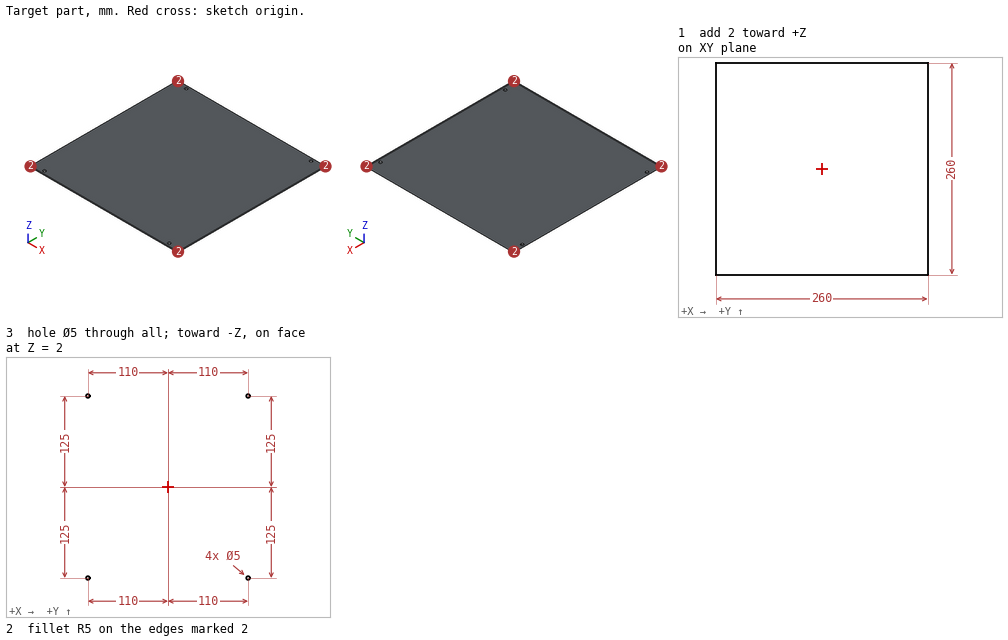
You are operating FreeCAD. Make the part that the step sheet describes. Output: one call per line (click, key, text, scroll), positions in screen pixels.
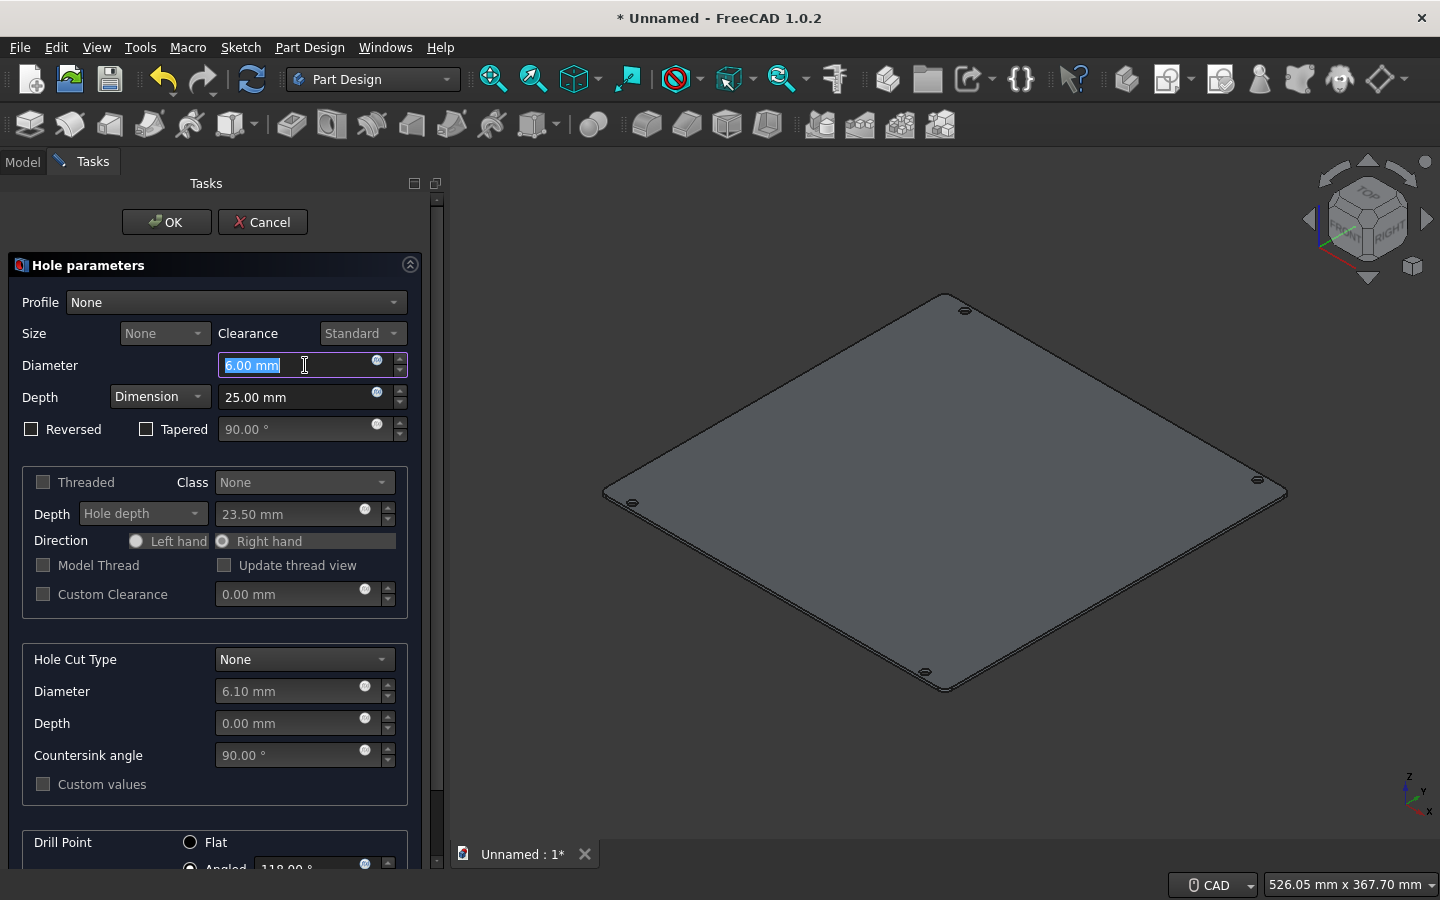
text(5)
key(Tab)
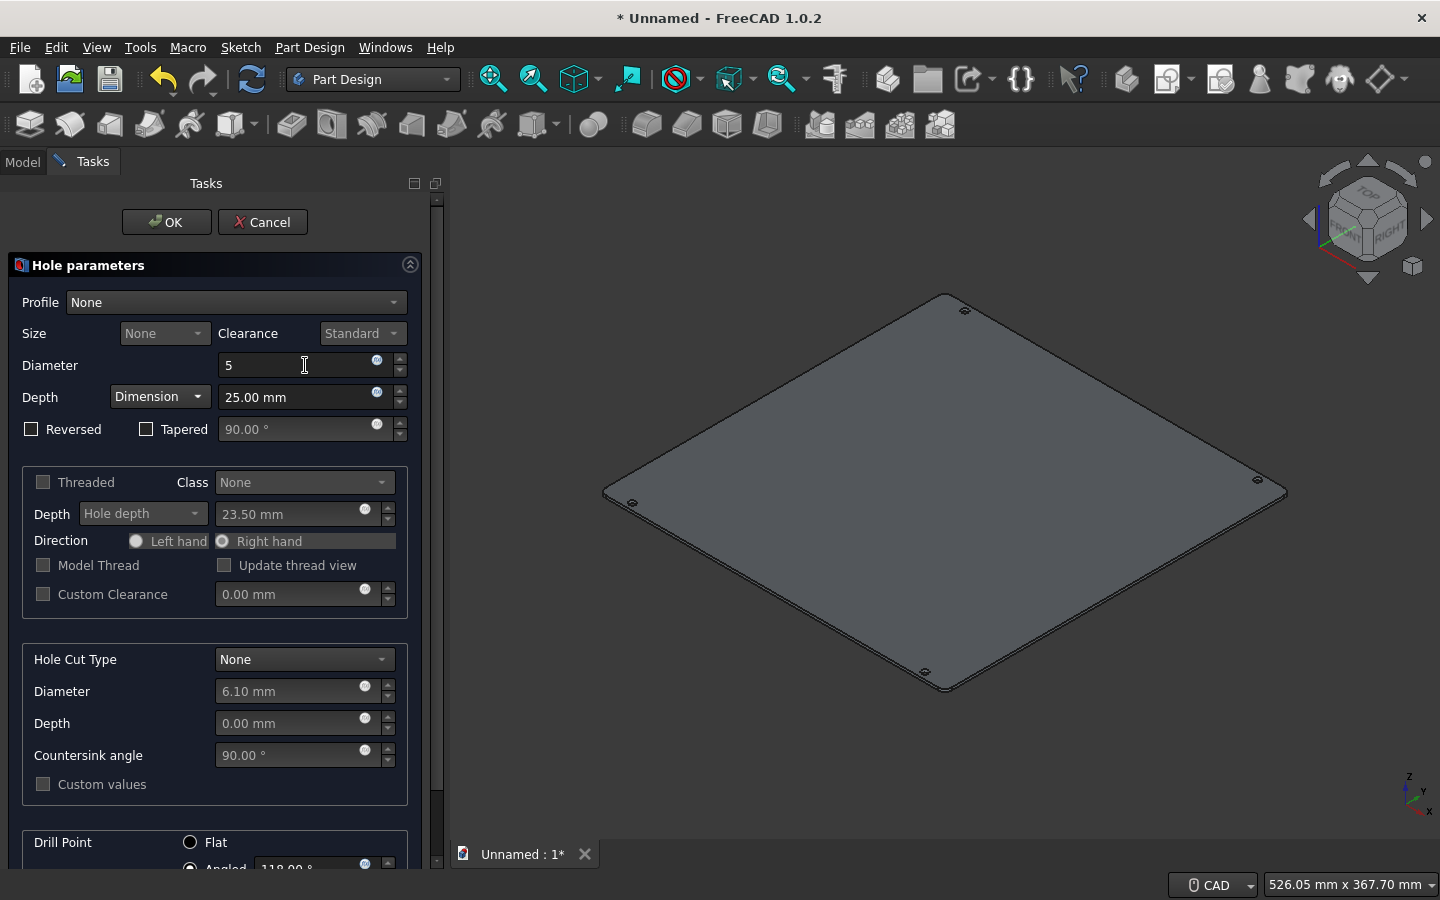
click(161, 396)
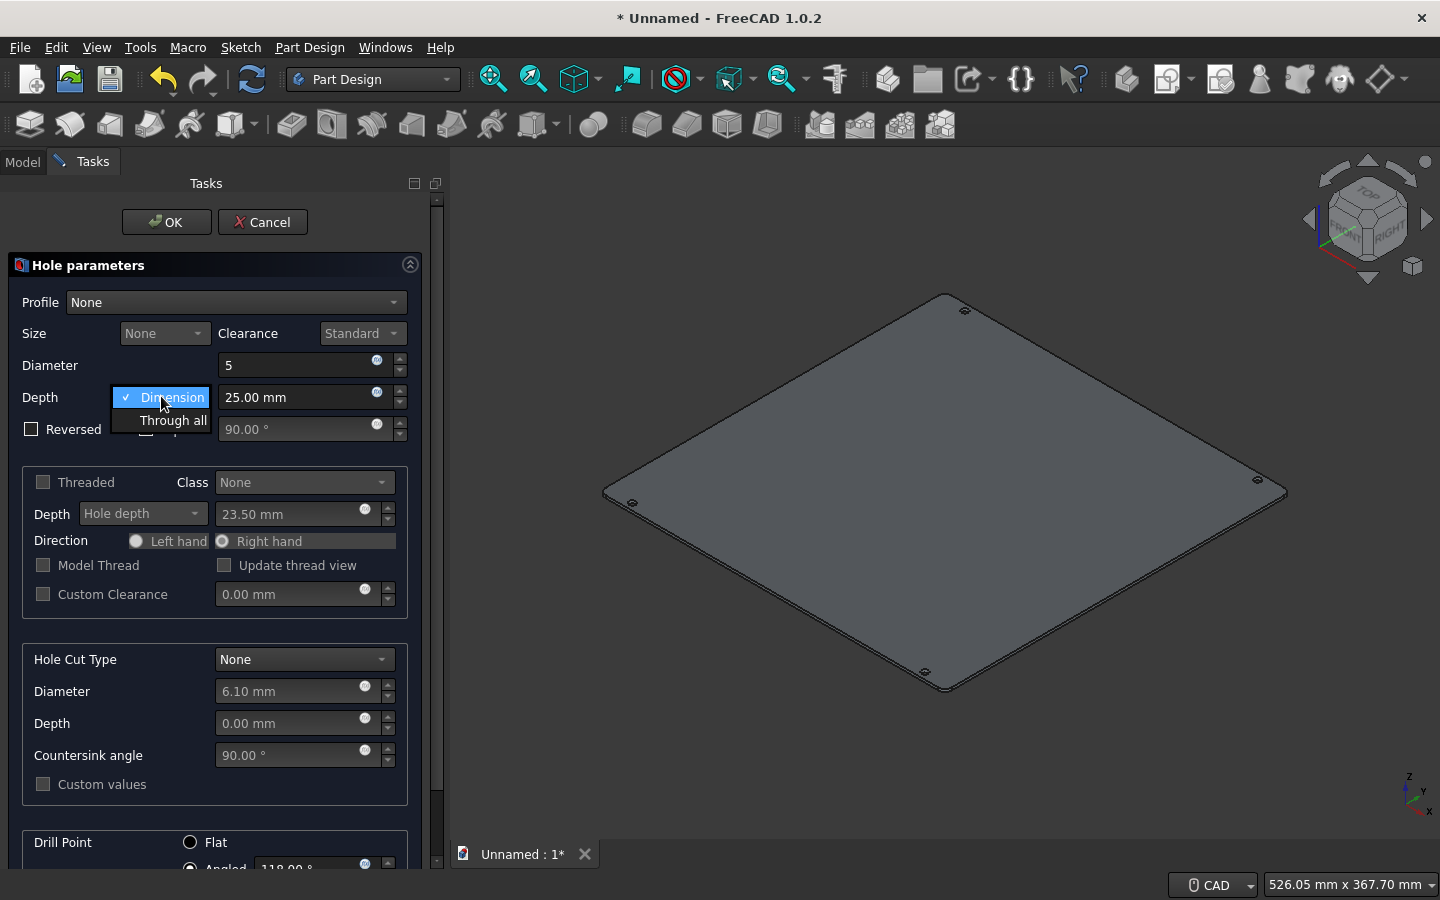
click(160, 420)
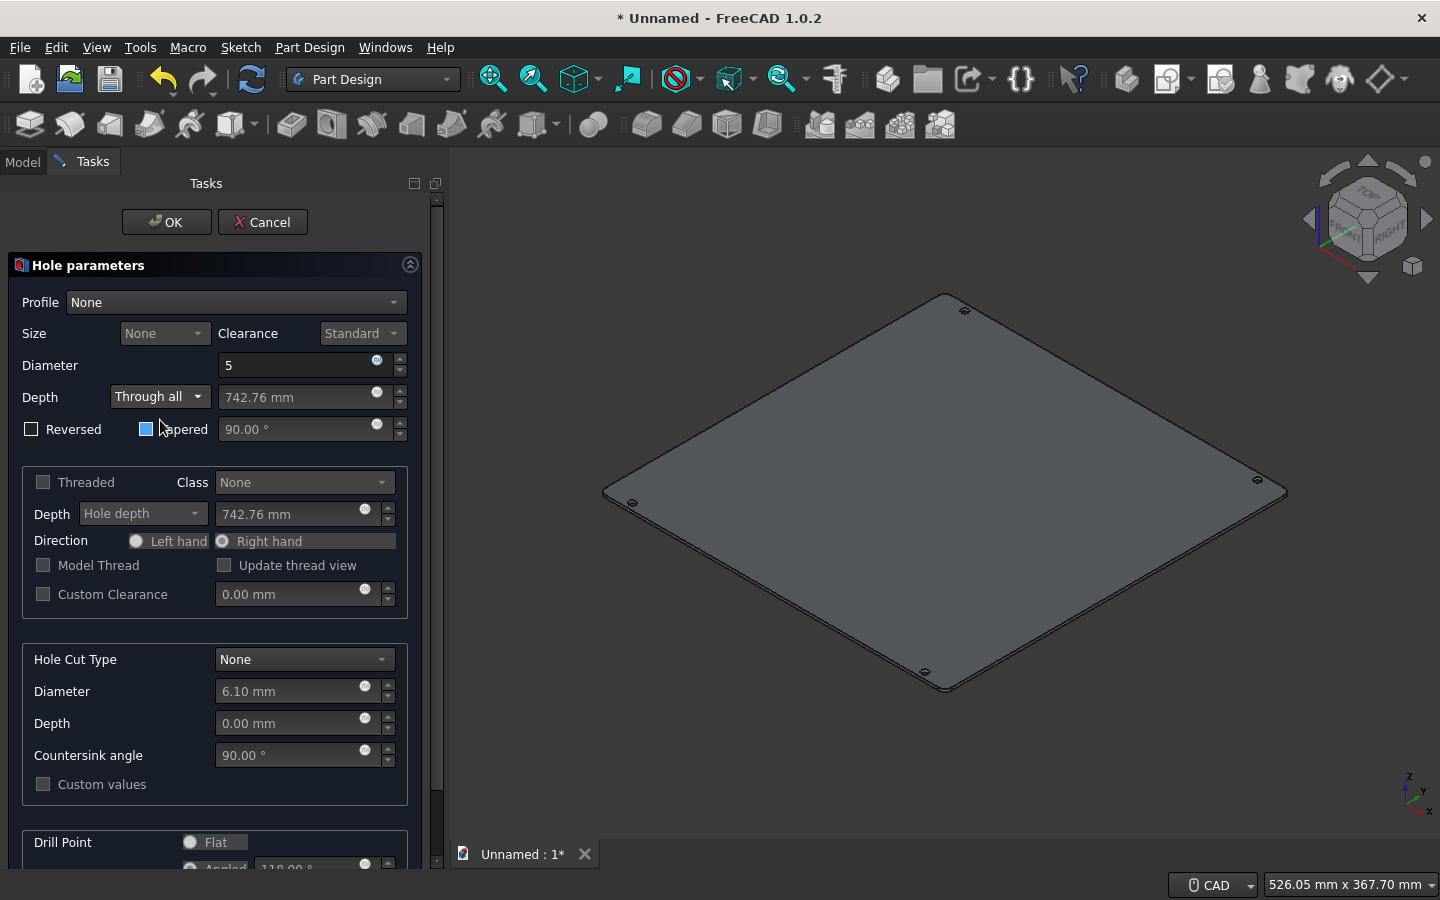
click(167, 222)